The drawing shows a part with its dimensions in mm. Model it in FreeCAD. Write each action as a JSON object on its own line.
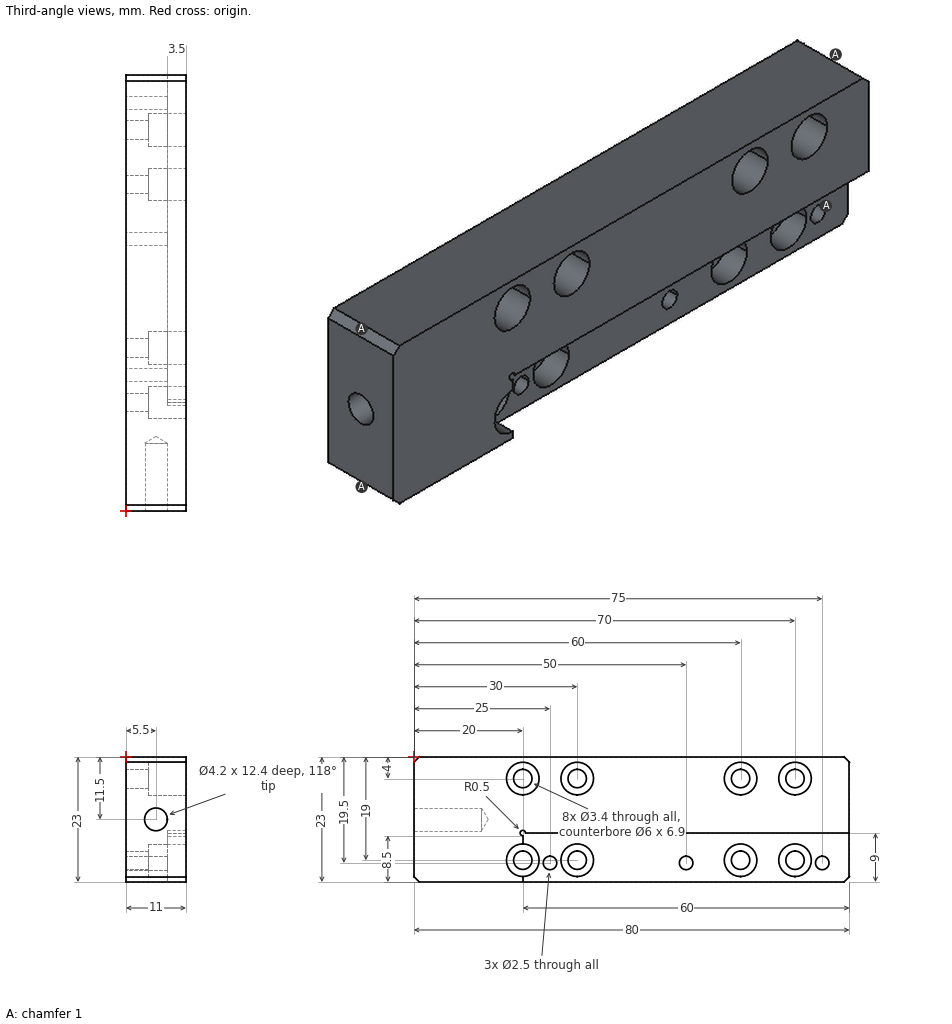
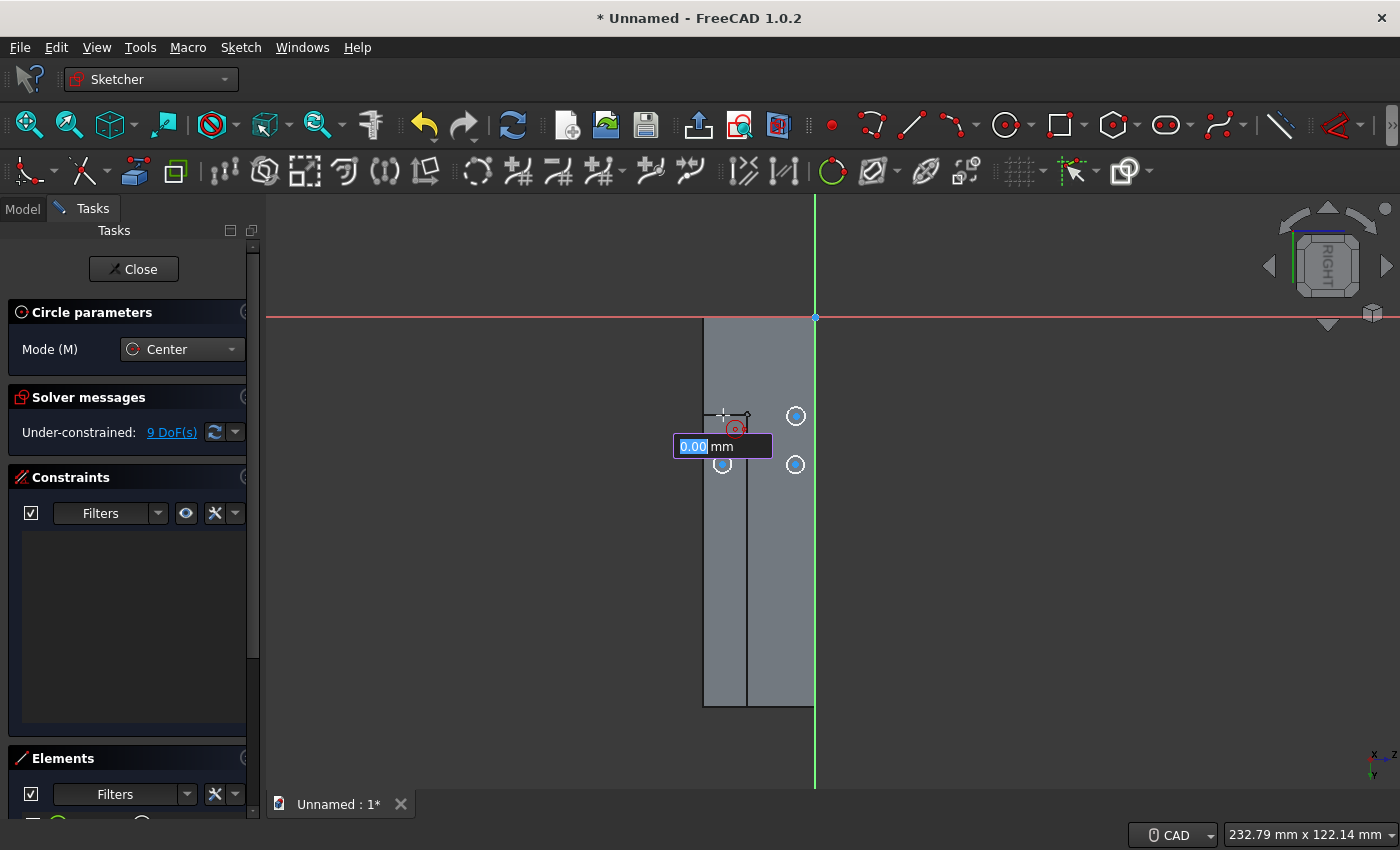
{"action": "scroll", "coordinate": [729, 409], "scroll_direction": "up", "scroll_amount": 4}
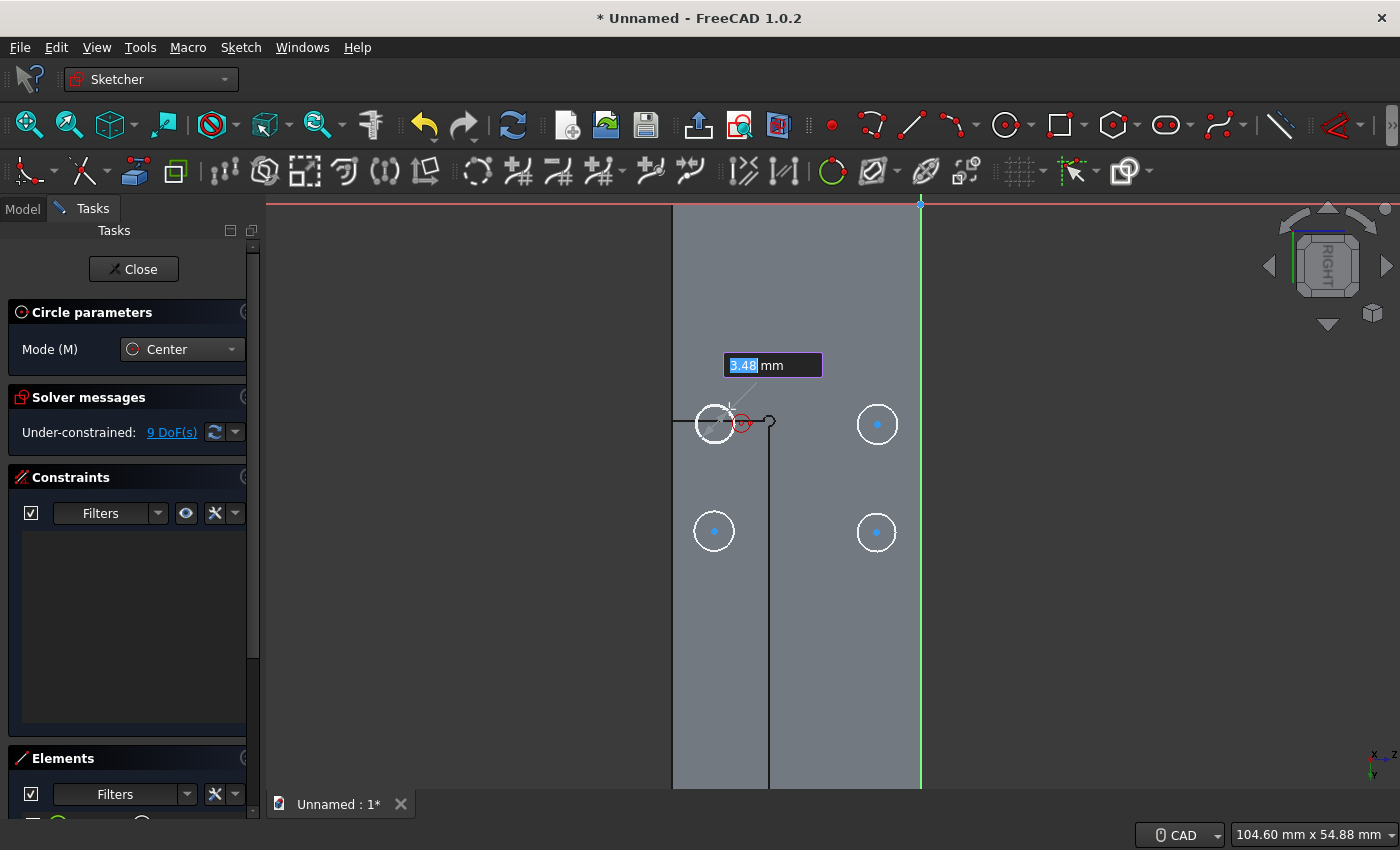
{"action": "left_click", "coordinate": [728, 408]}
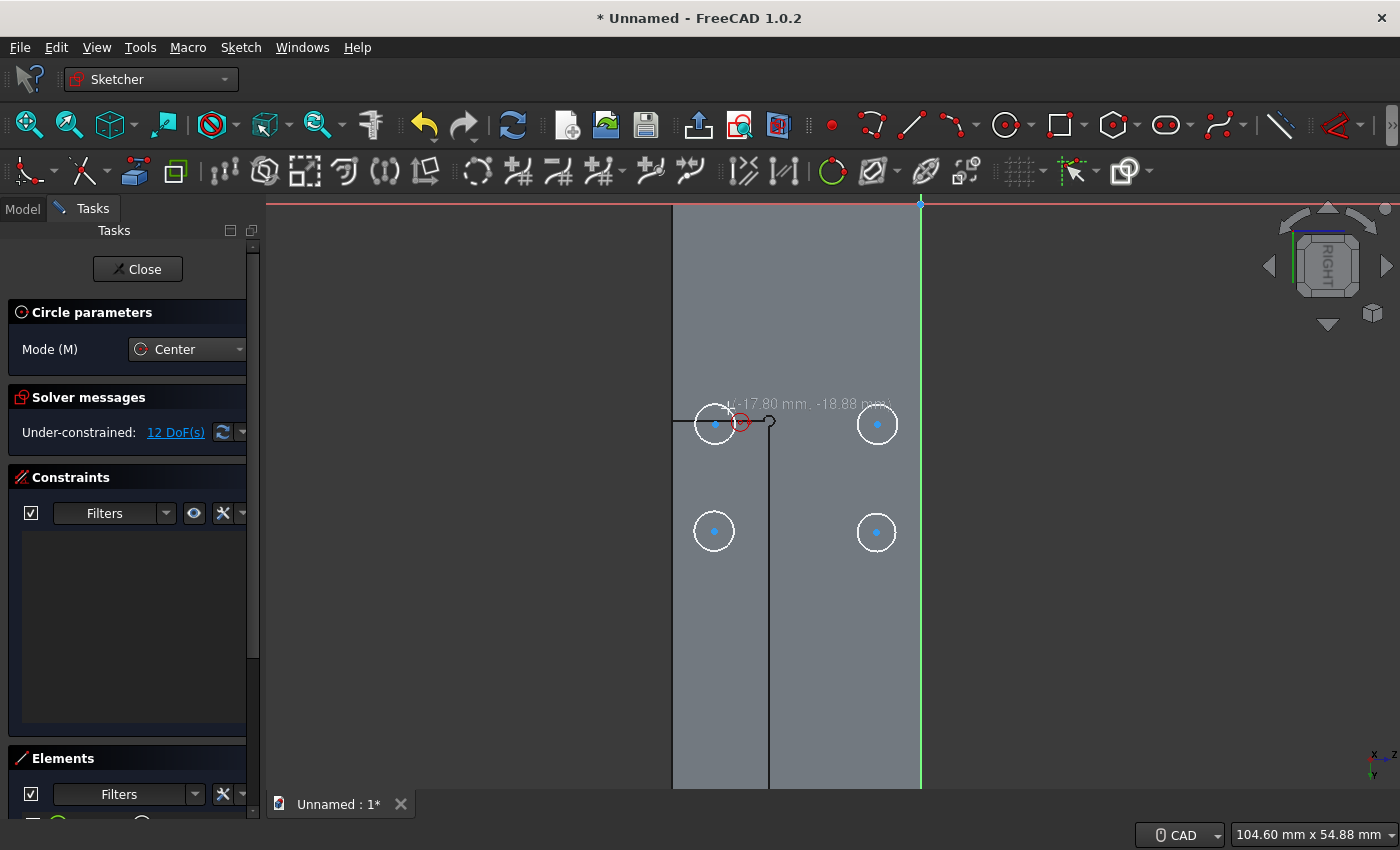
{"action": "scroll", "coordinate": [728, 409], "scroll_direction": "down", "scroll_amount": 4}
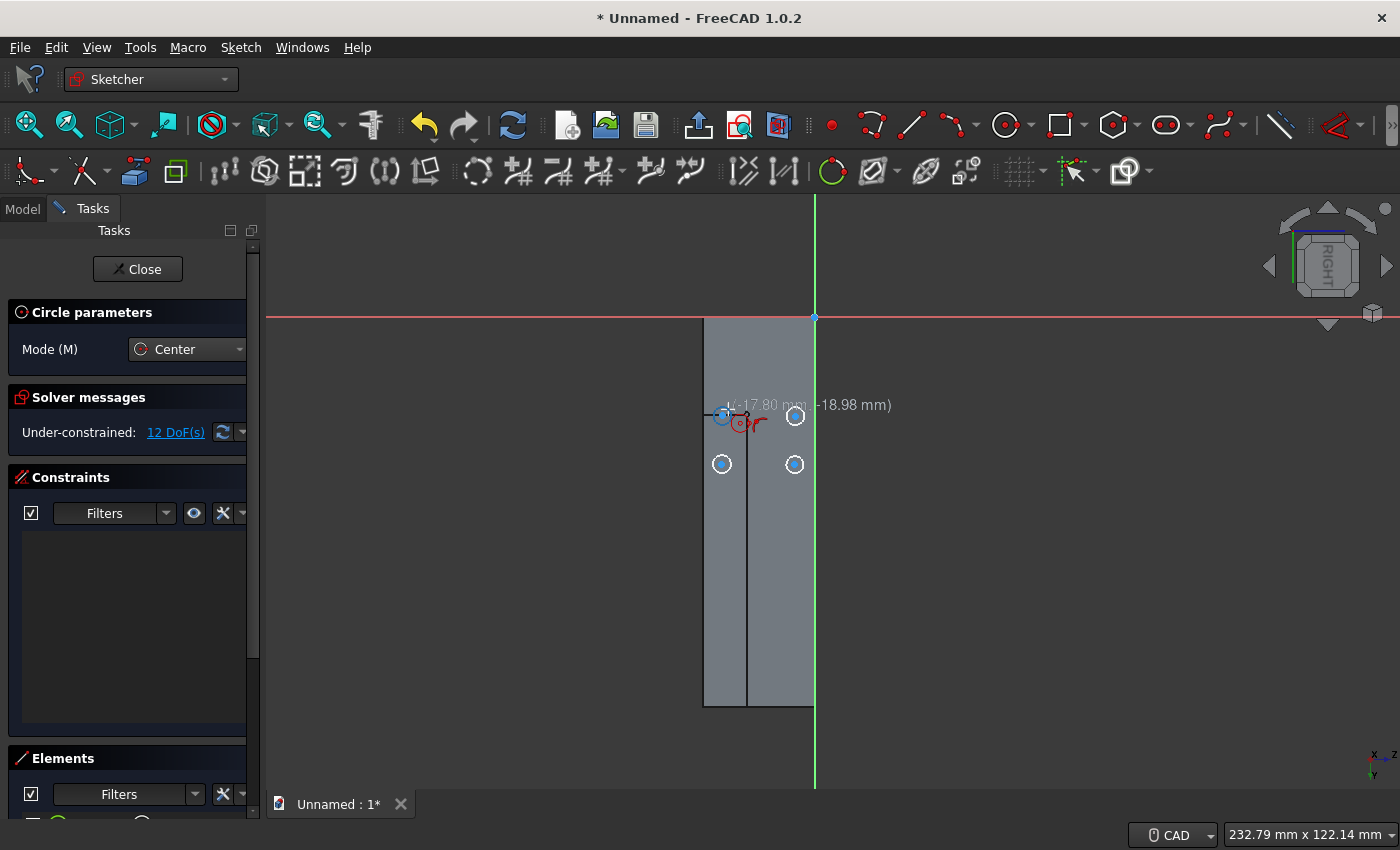
{"action": "scroll", "coordinate": [795, 609], "scroll_direction": "up", "scroll_amount": 6}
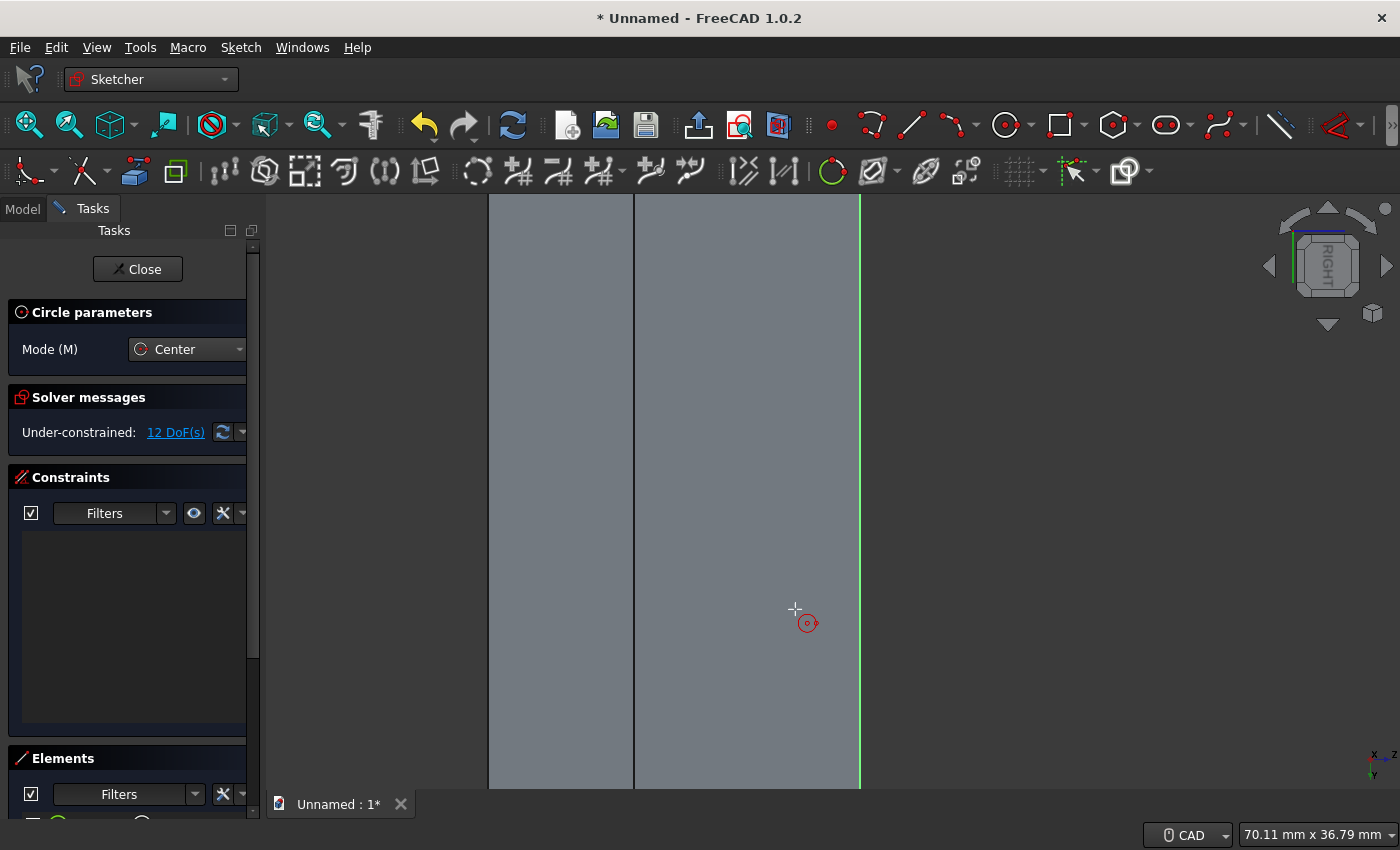
{"action": "scroll", "coordinate": [795, 609], "scroll_direction": "down", "scroll_amount": 6}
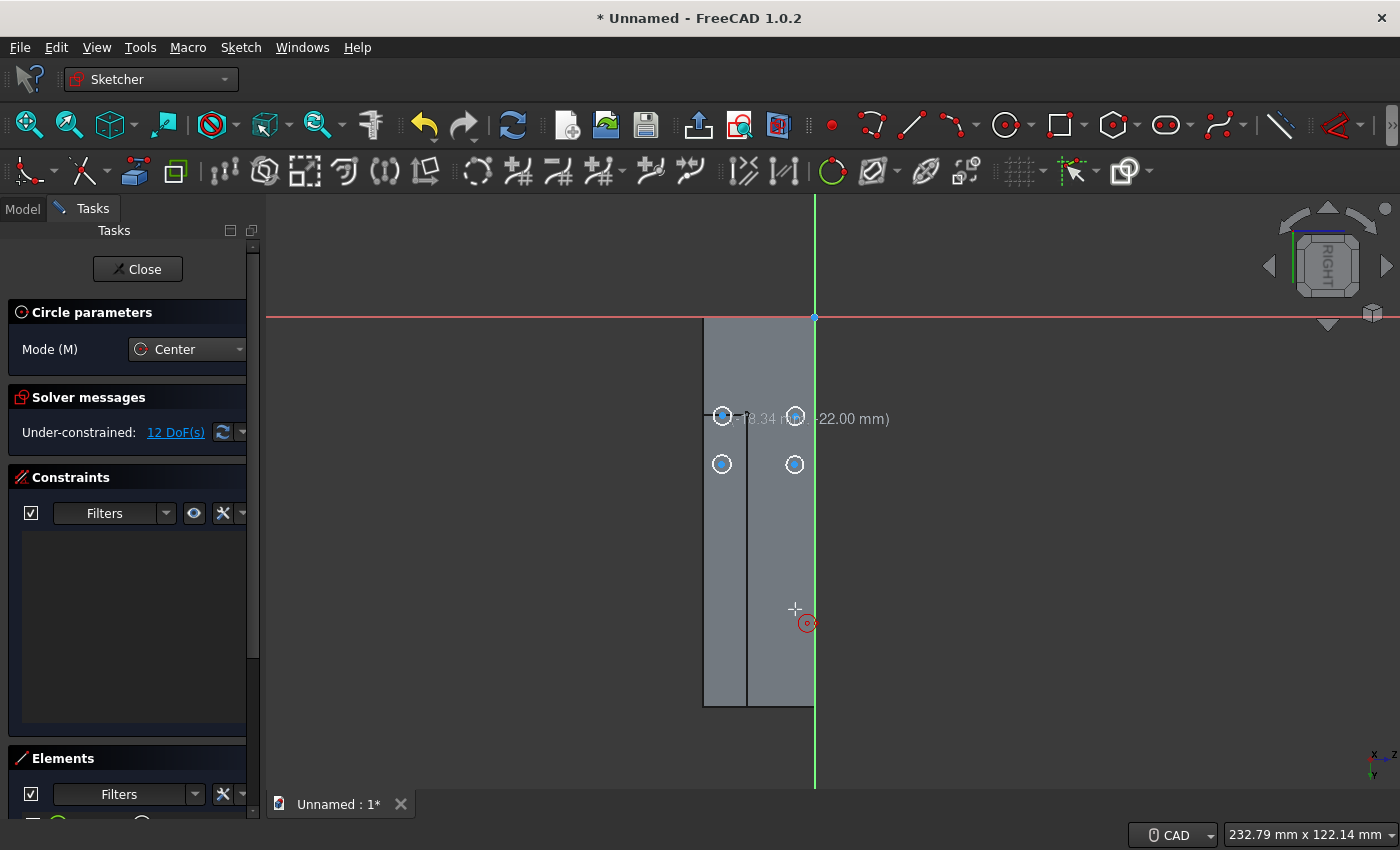
{"action": "left_click", "coordinate": [795, 609]}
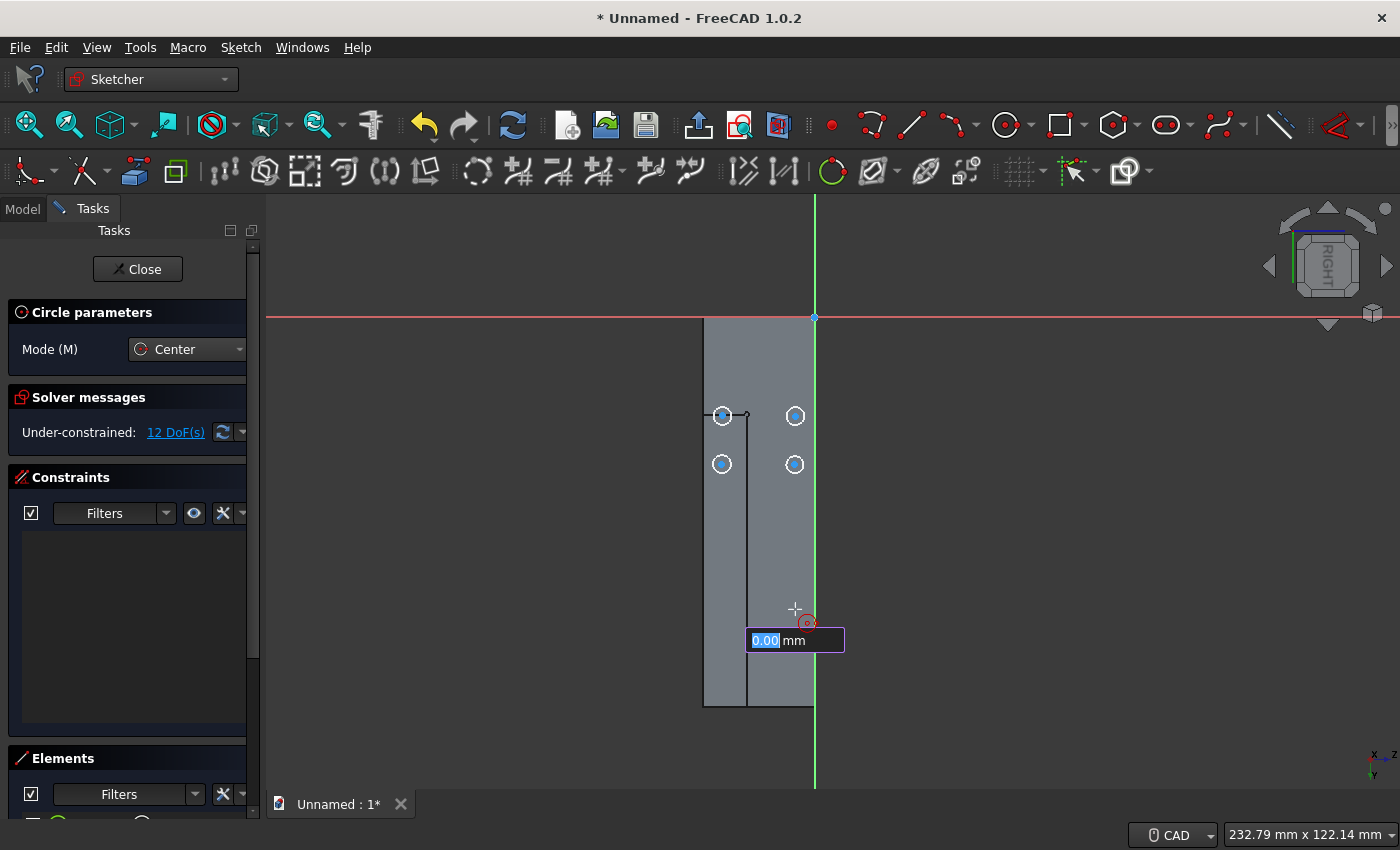
{"action": "scroll", "coordinate": [790, 604], "scroll_direction": "up", "scroll_amount": 4}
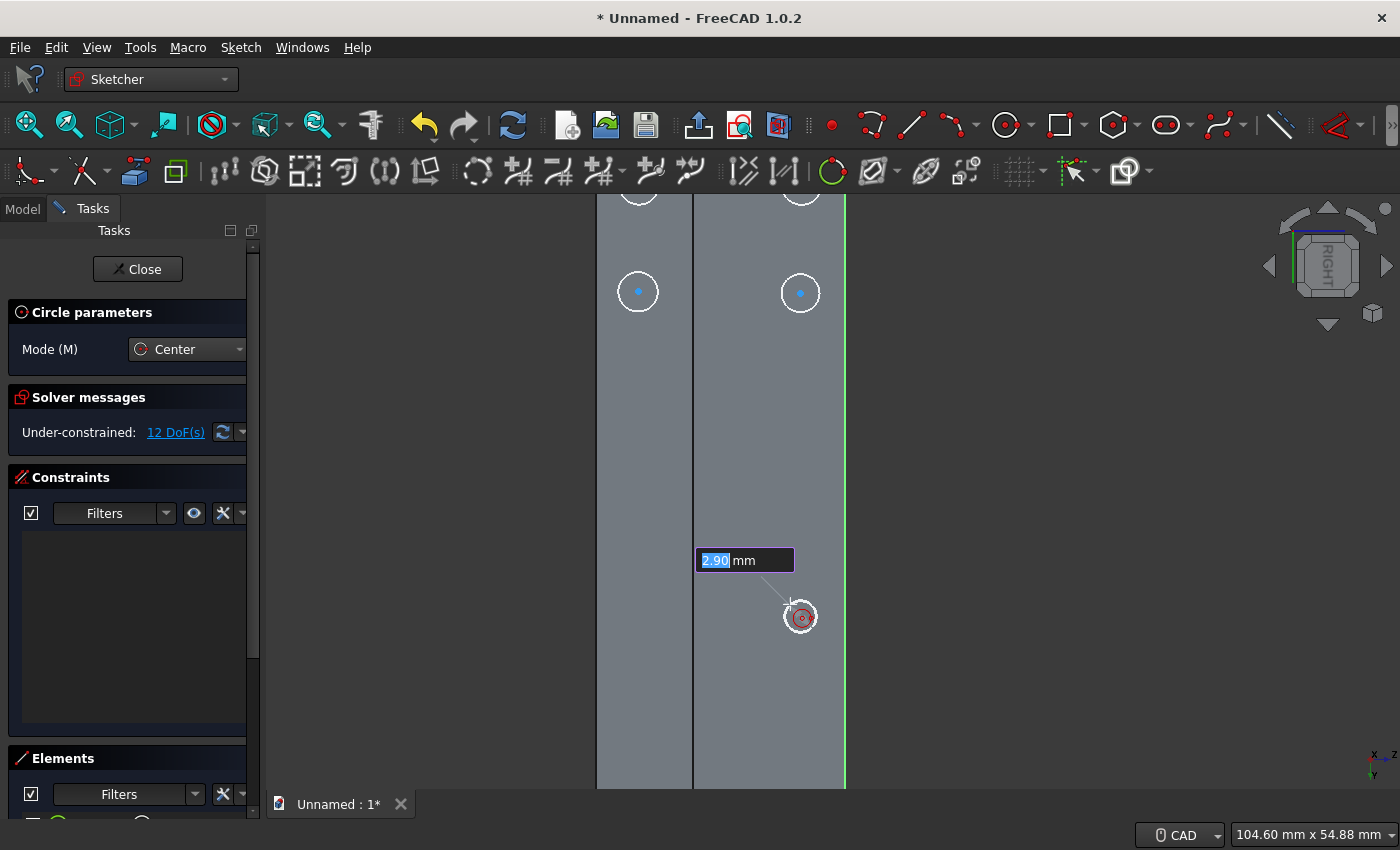
{"action": "left_click", "coordinate": [788, 602]}